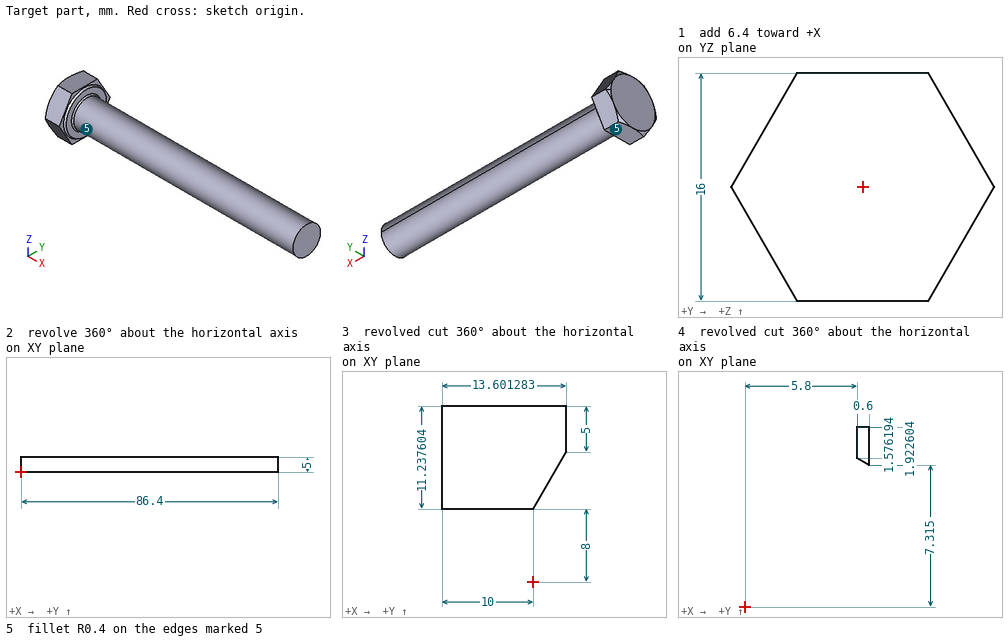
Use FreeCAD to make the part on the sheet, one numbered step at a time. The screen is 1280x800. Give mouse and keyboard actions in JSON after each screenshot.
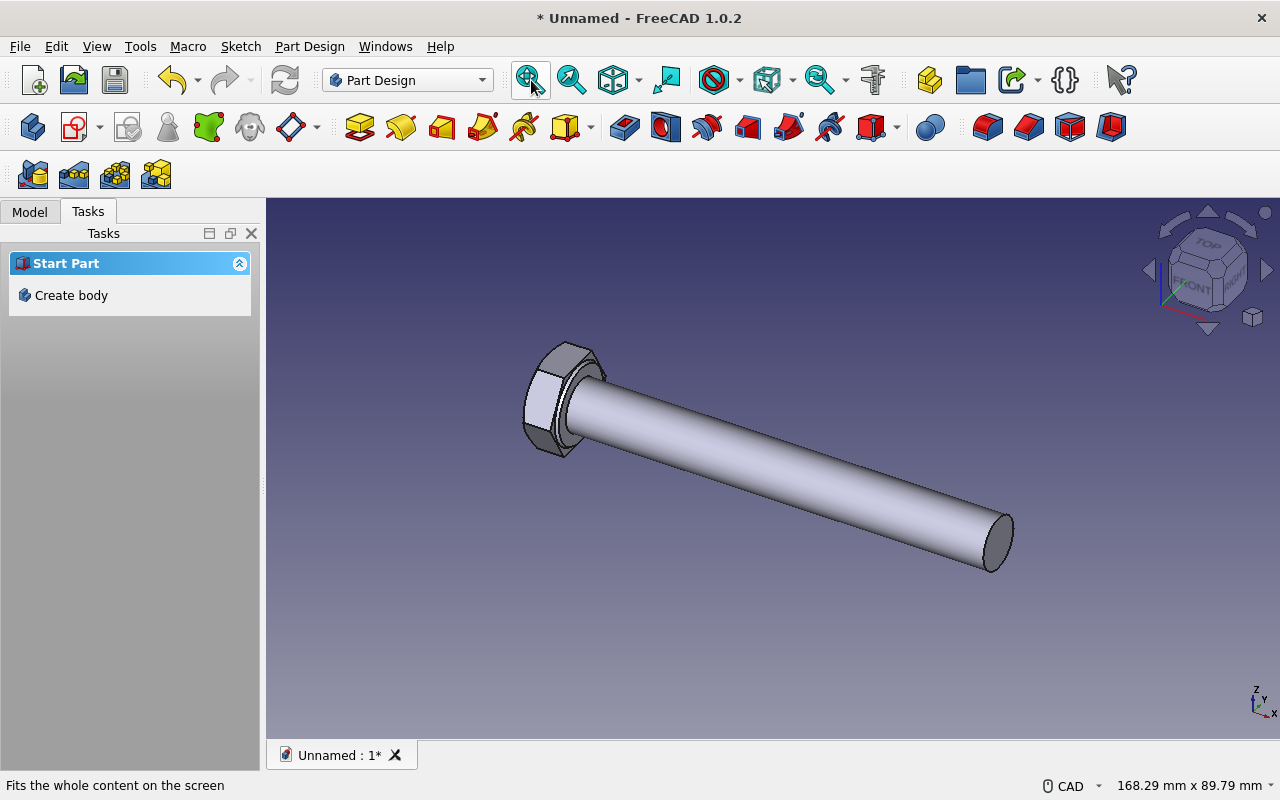
{"action": "key", "text": "0"}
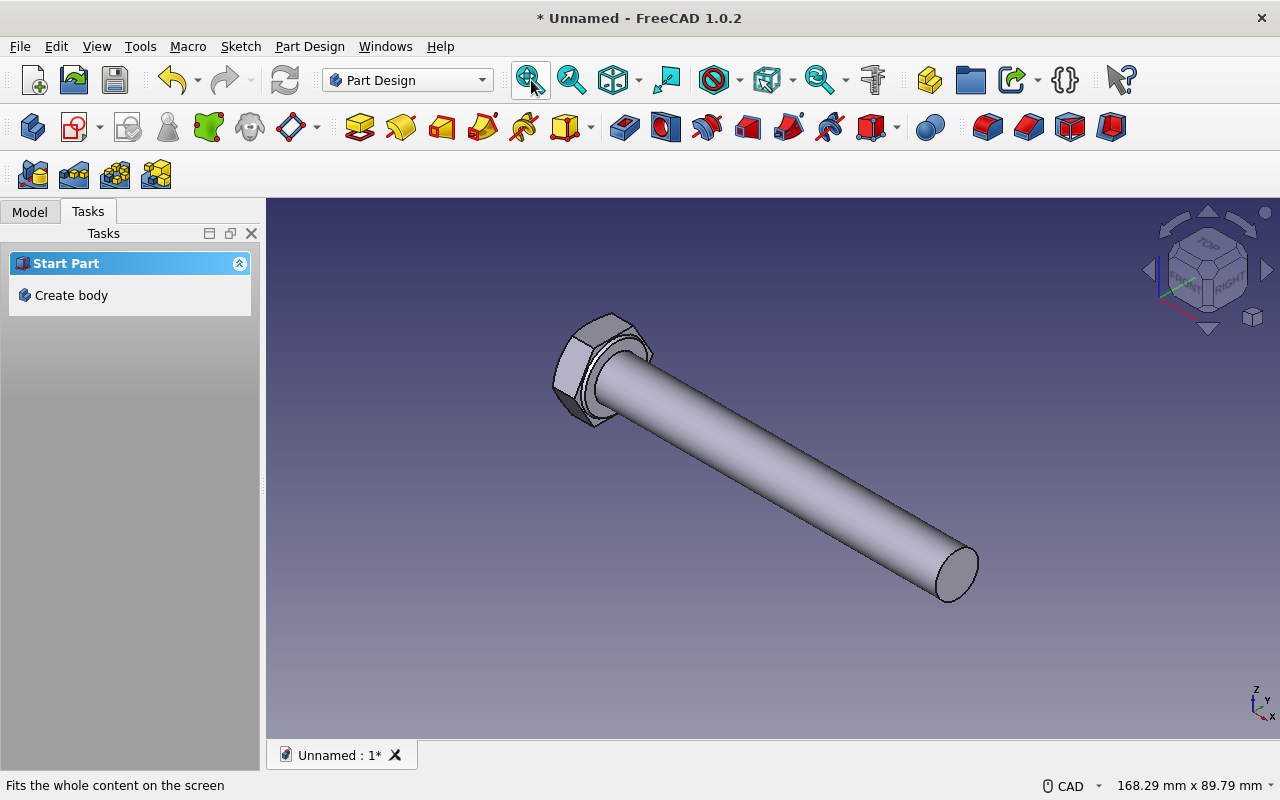
{"action": "key", "text": "2"}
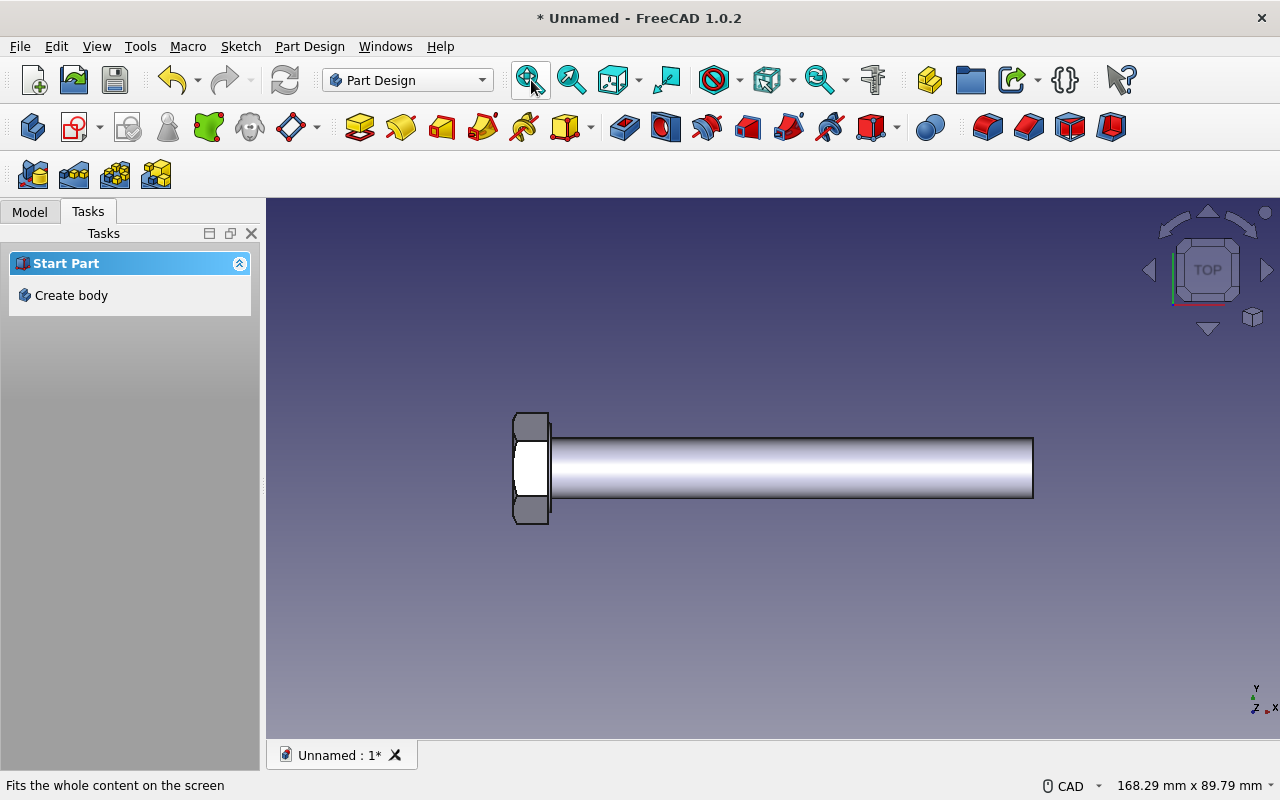
{"action": "key", "text": "1"}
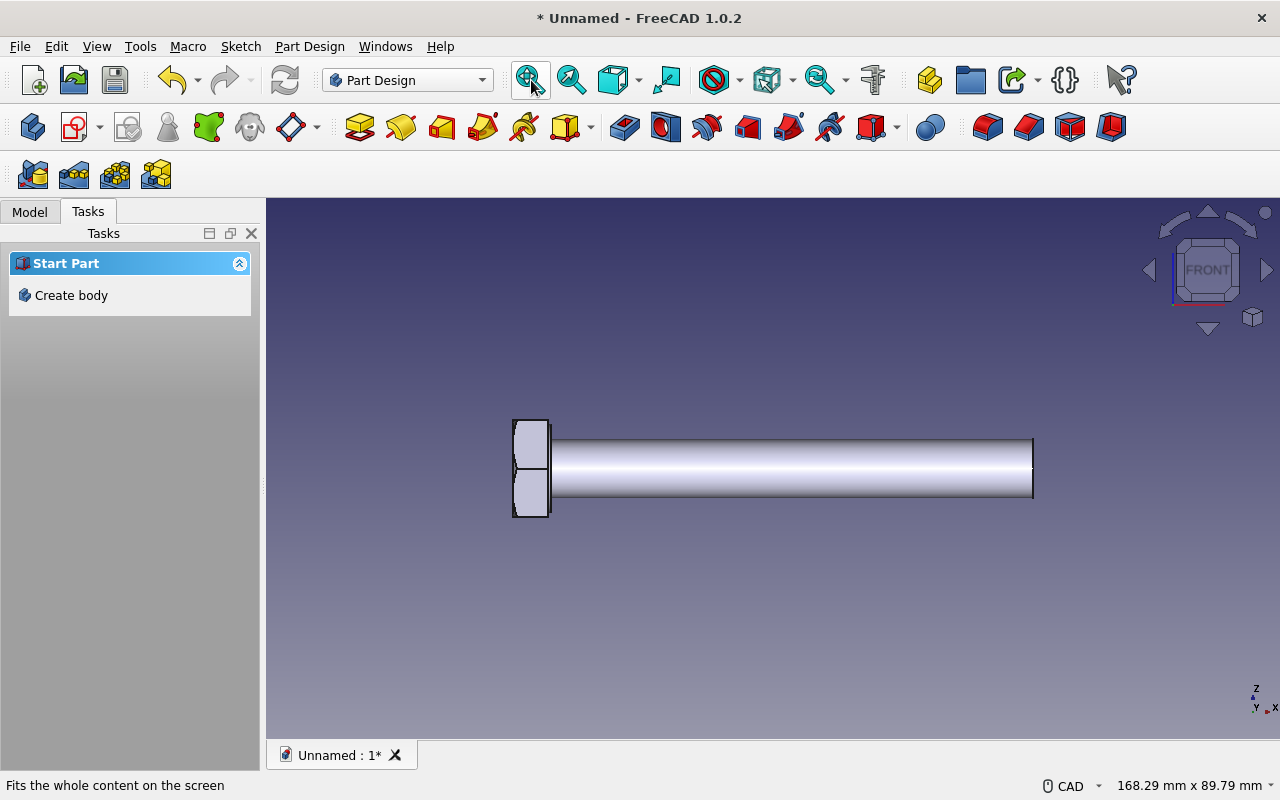
{"action": "key", "text": "3"}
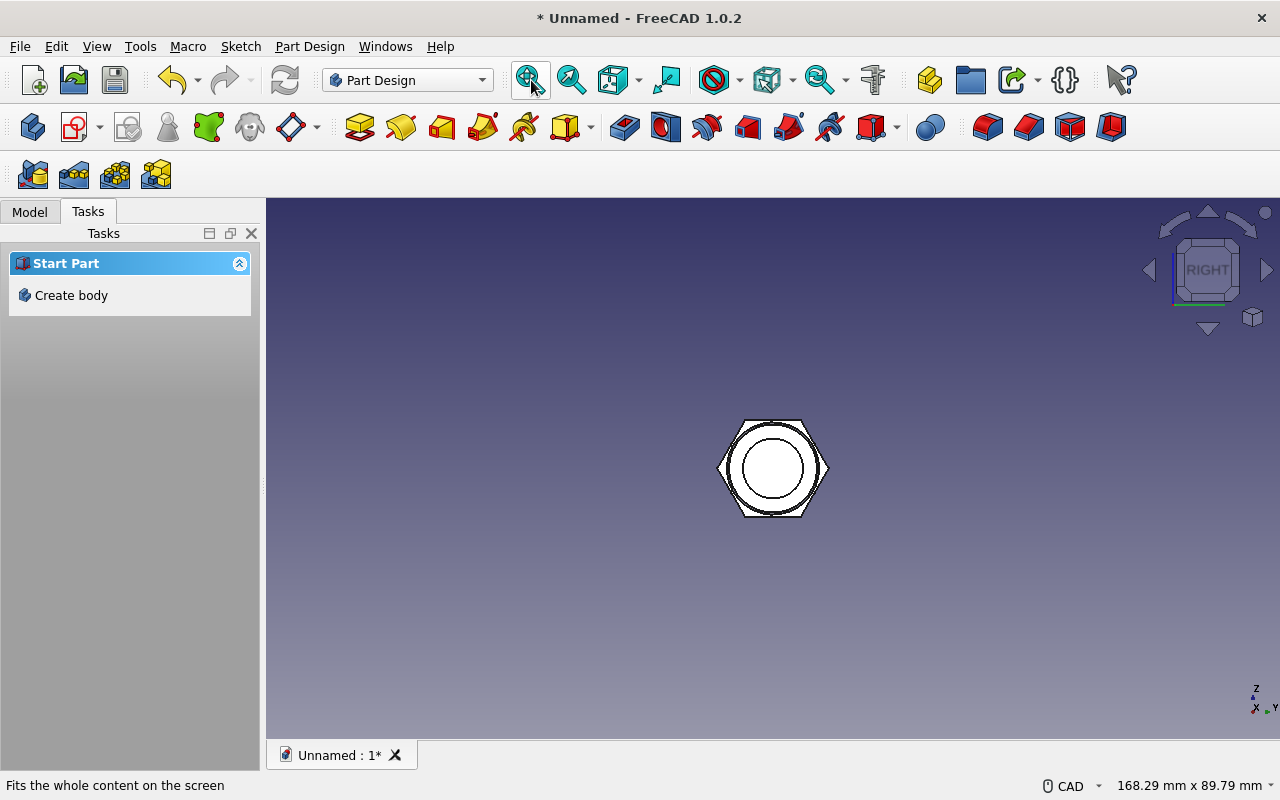
{"action": "left_click", "coordinate": [531, 80]}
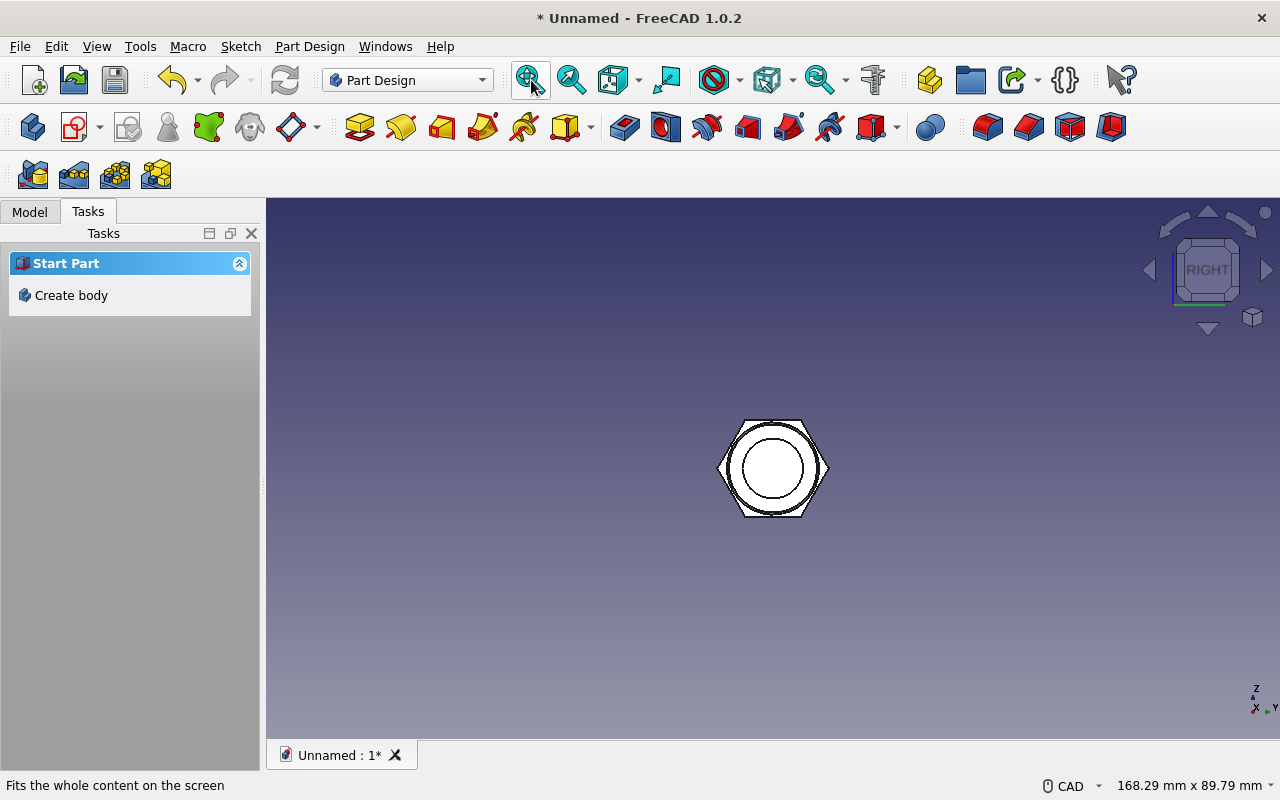
{"action": "key", "text": "5"}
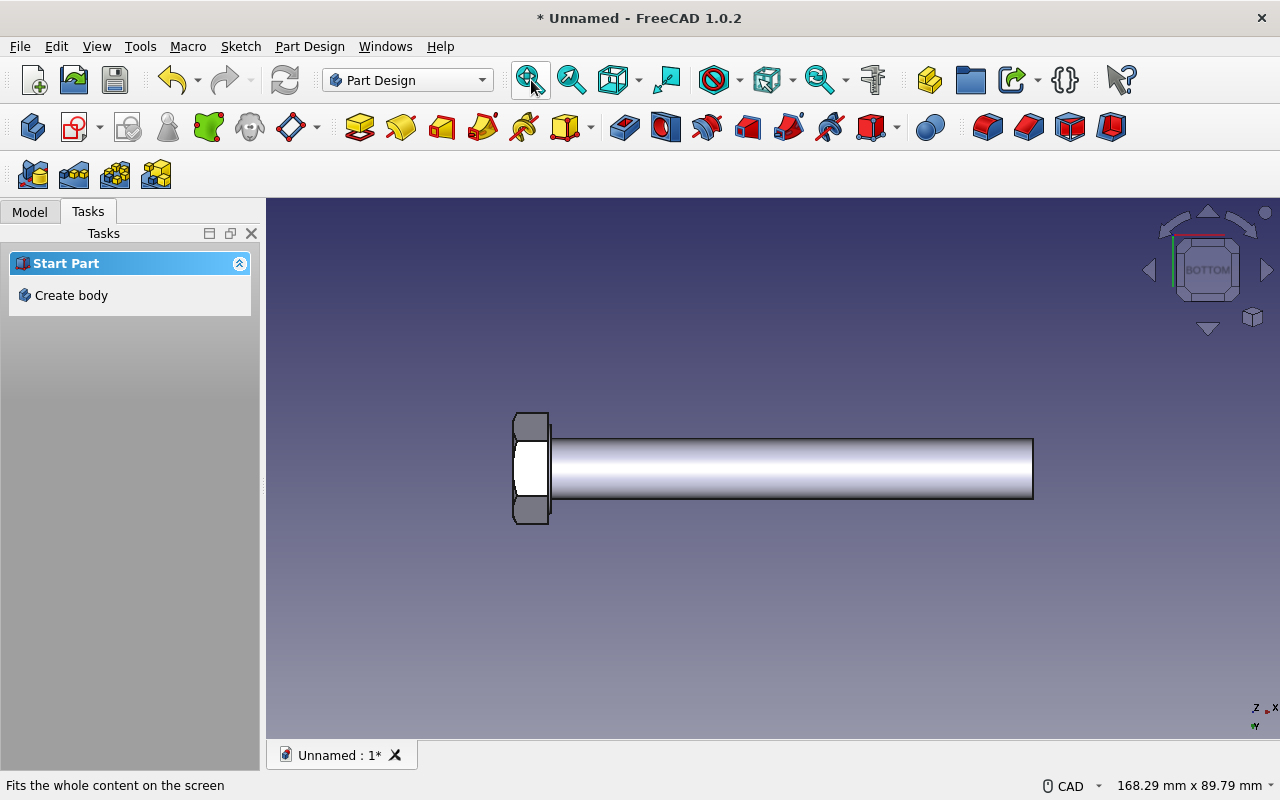
{"action": "key", "text": "4"}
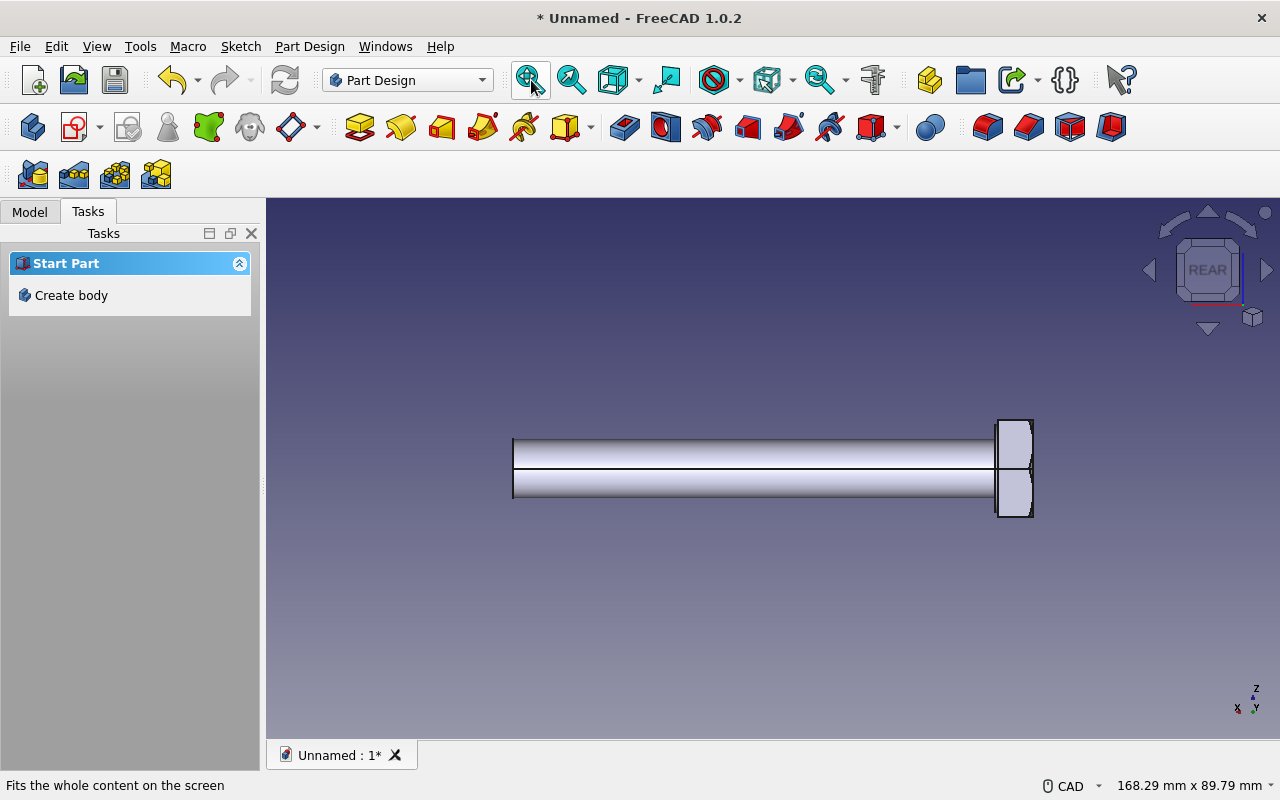
{"action": "key", "text": "6"}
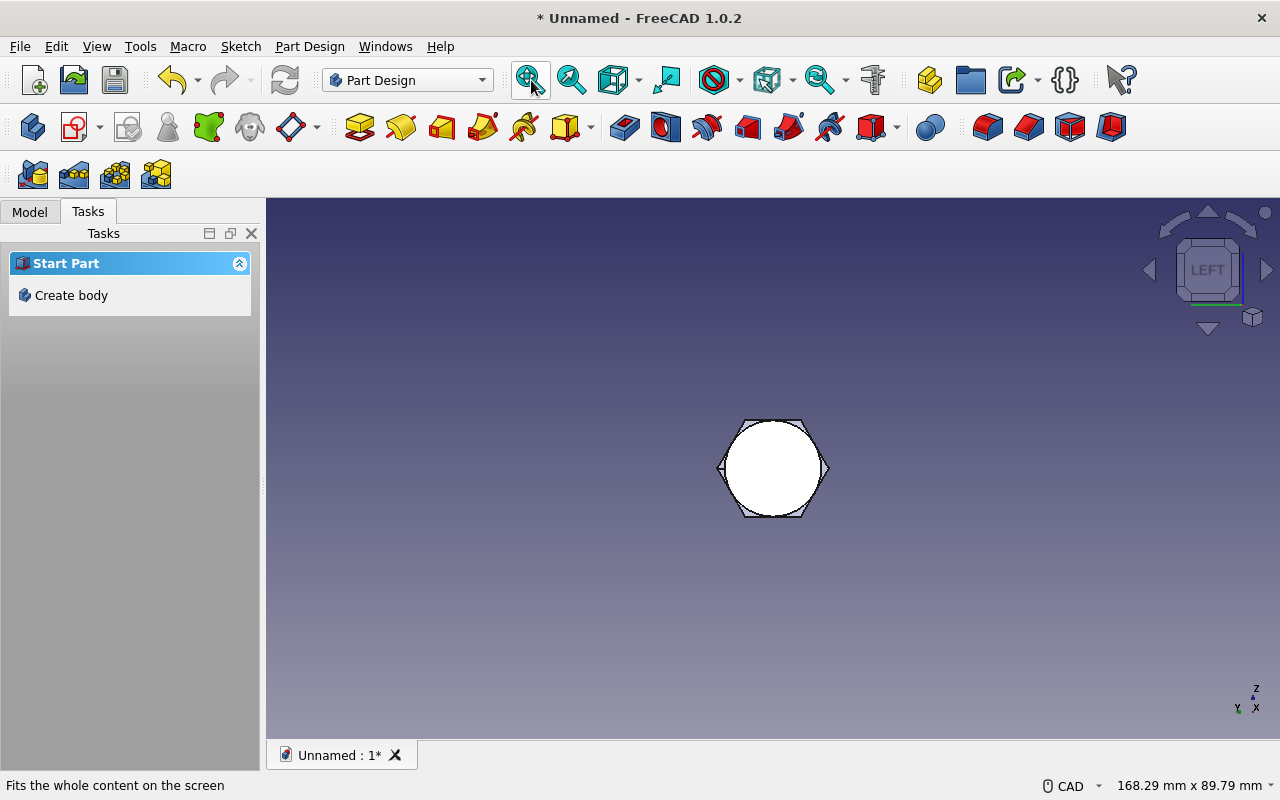
{"action": "left_click", "coordinate": [531, 80]}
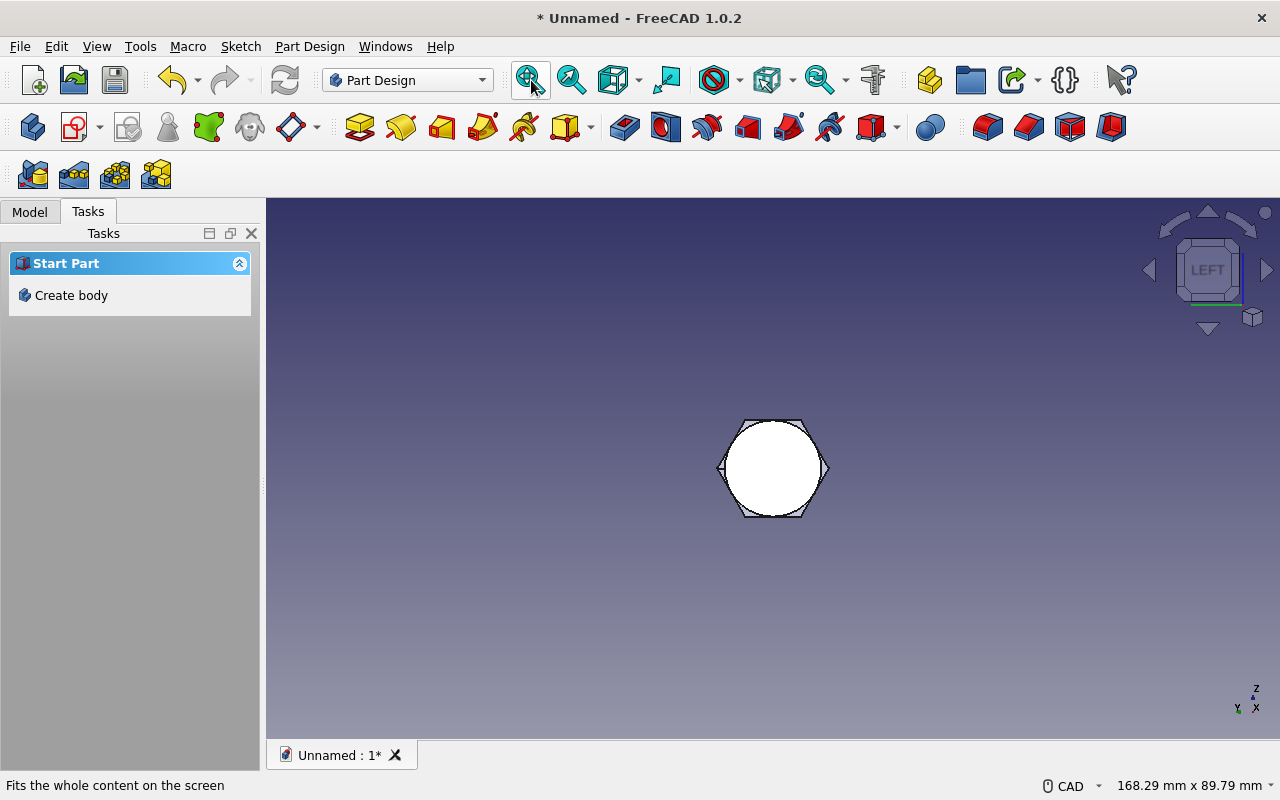
{"action": "key", "text": "v 3"}